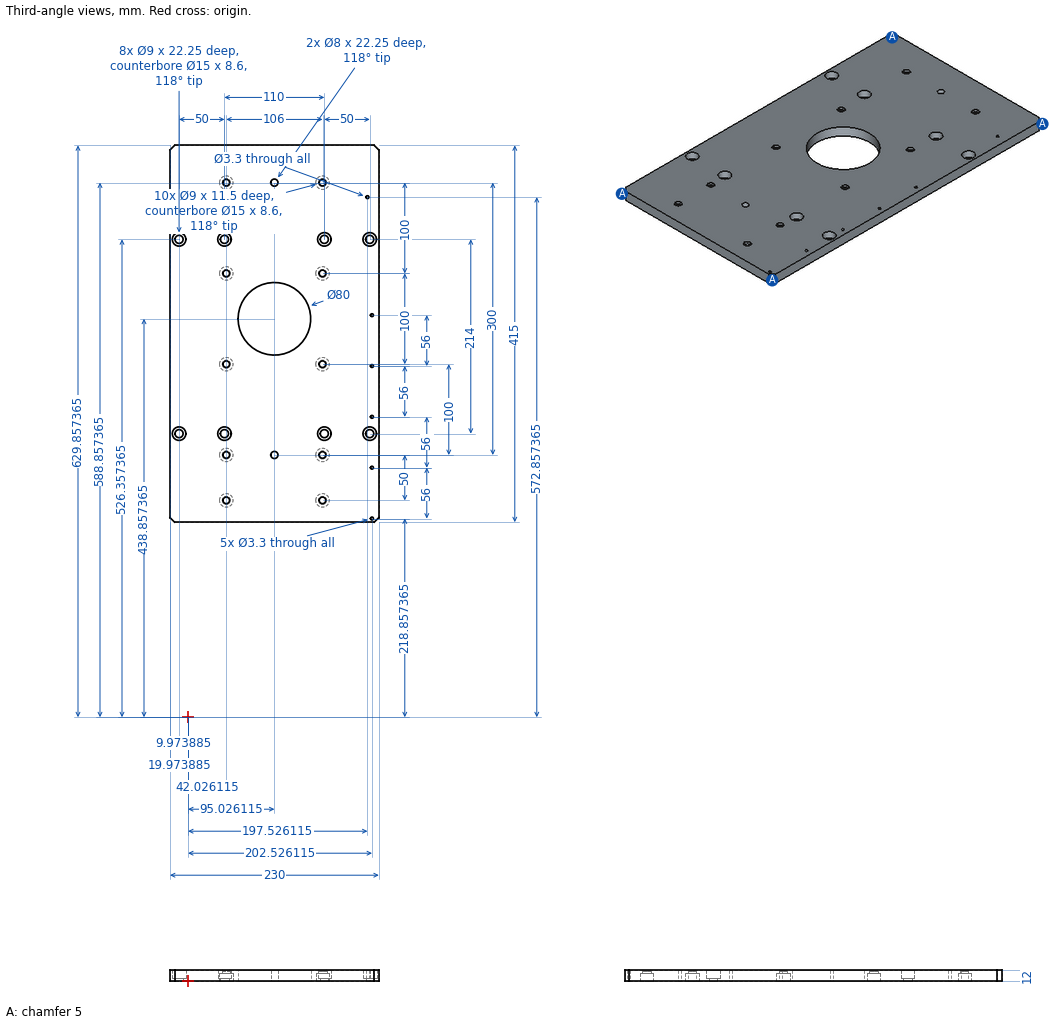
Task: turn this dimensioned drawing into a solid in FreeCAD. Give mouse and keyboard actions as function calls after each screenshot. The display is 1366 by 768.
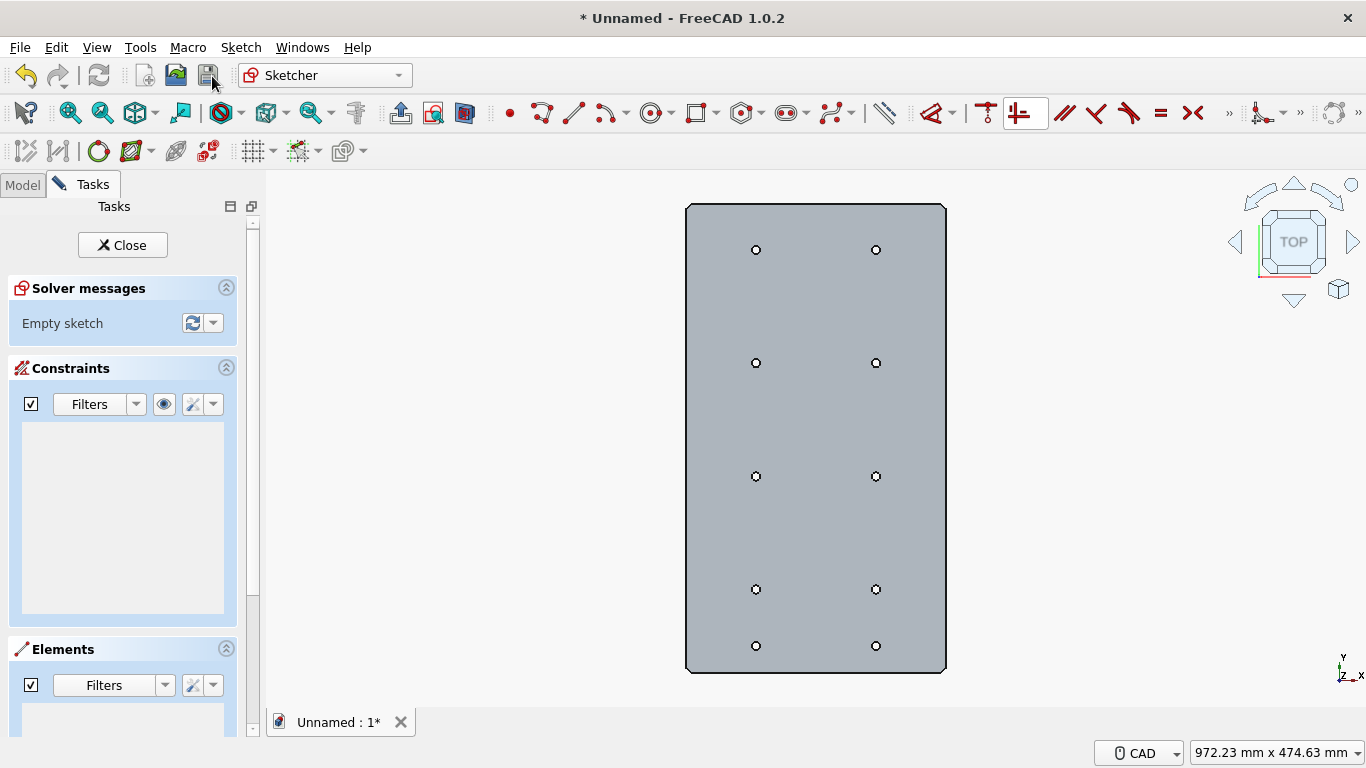
scroll(664, 223, down, 3)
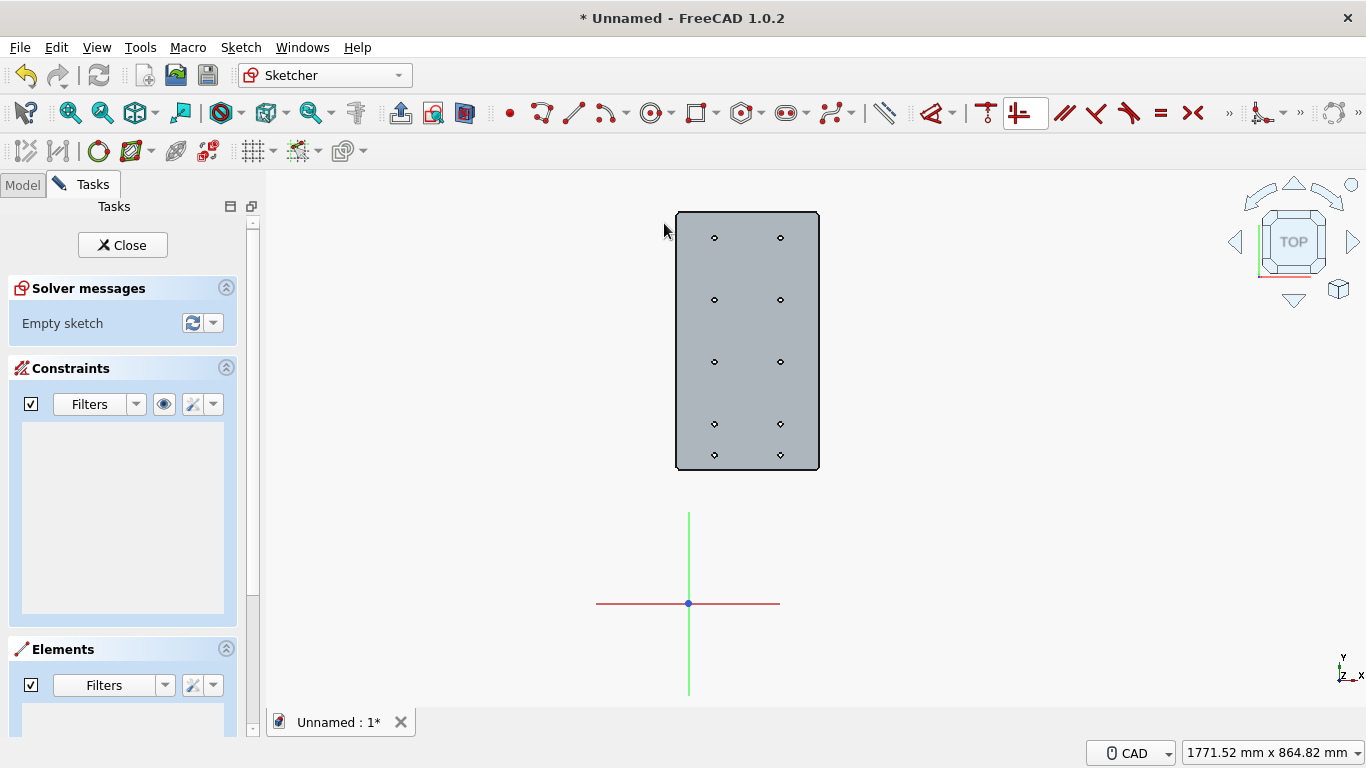
click(652, 114)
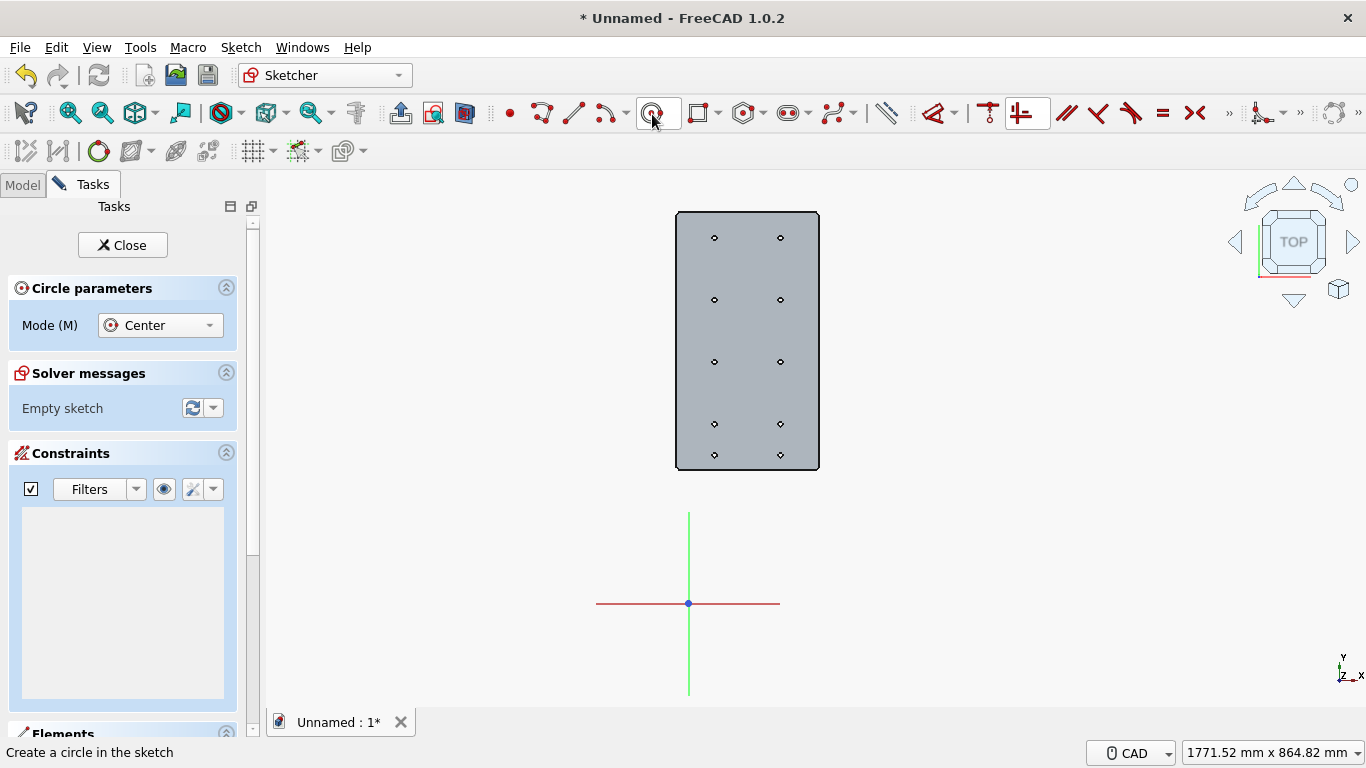
scroll(682, 277, up, 11)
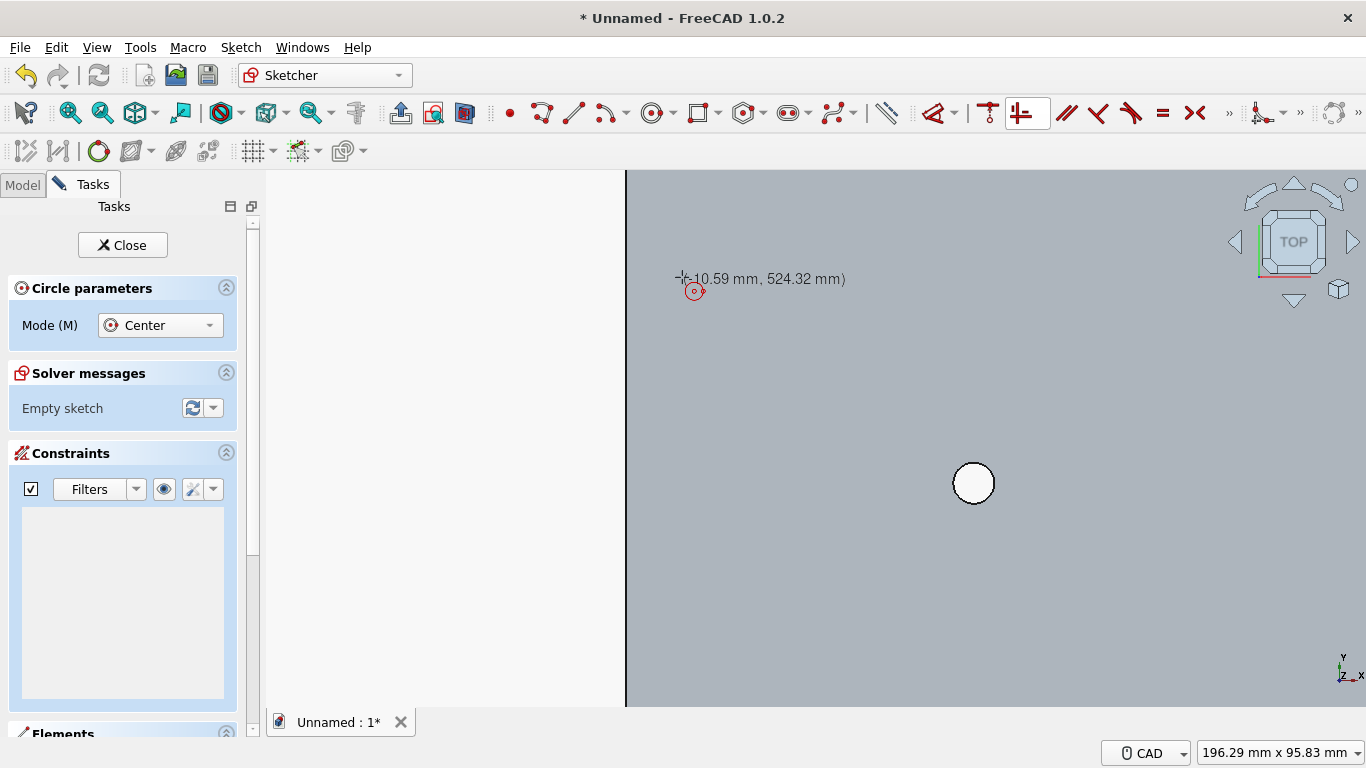
scroll(682, 277, down, 11)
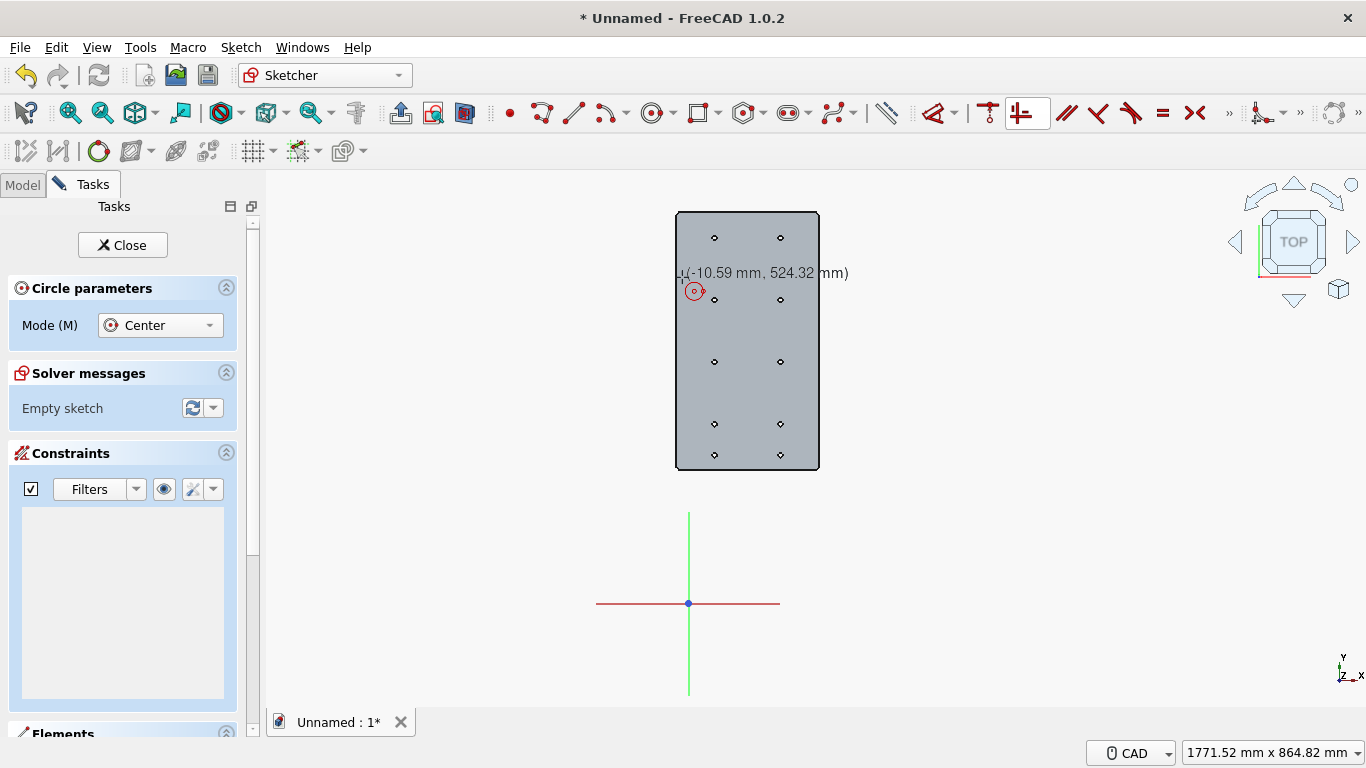
scroll(682, 277, up, 5)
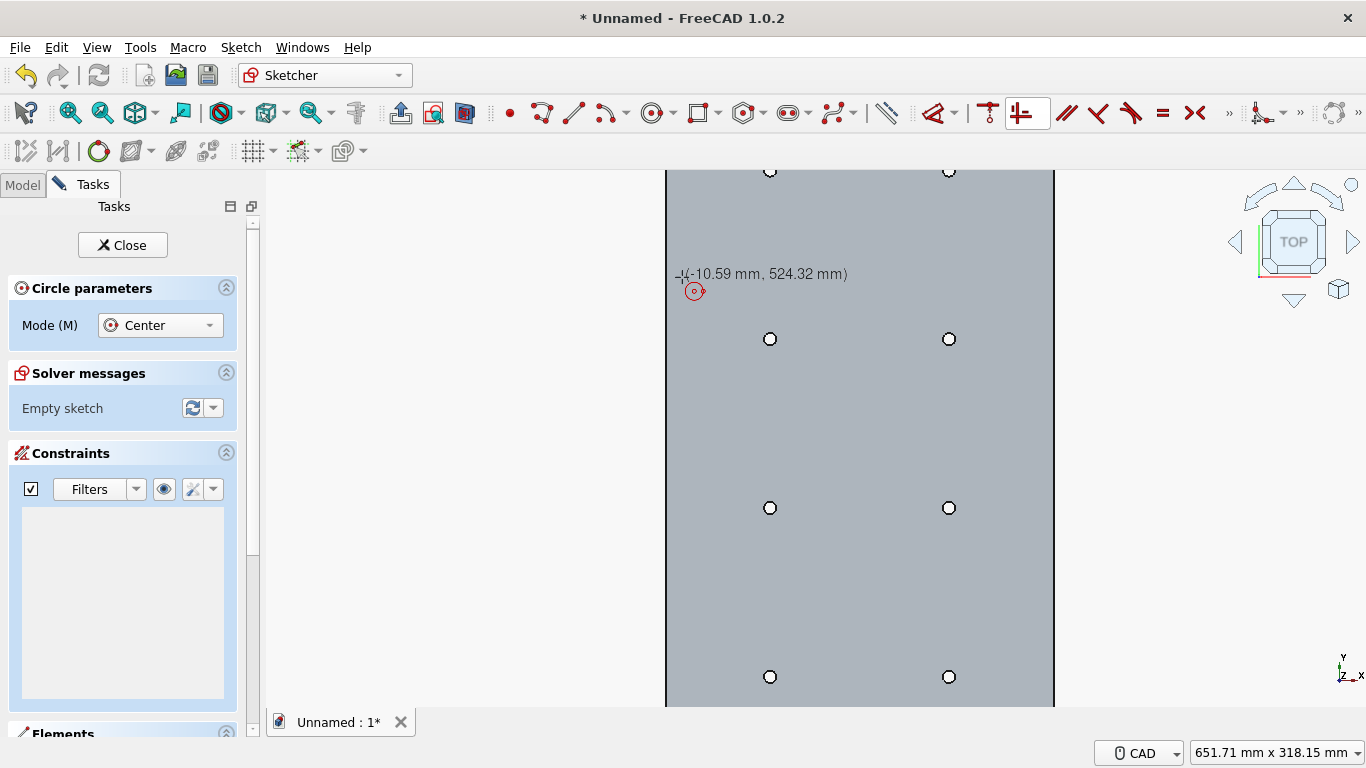
click(682, 276)
move(677, 271)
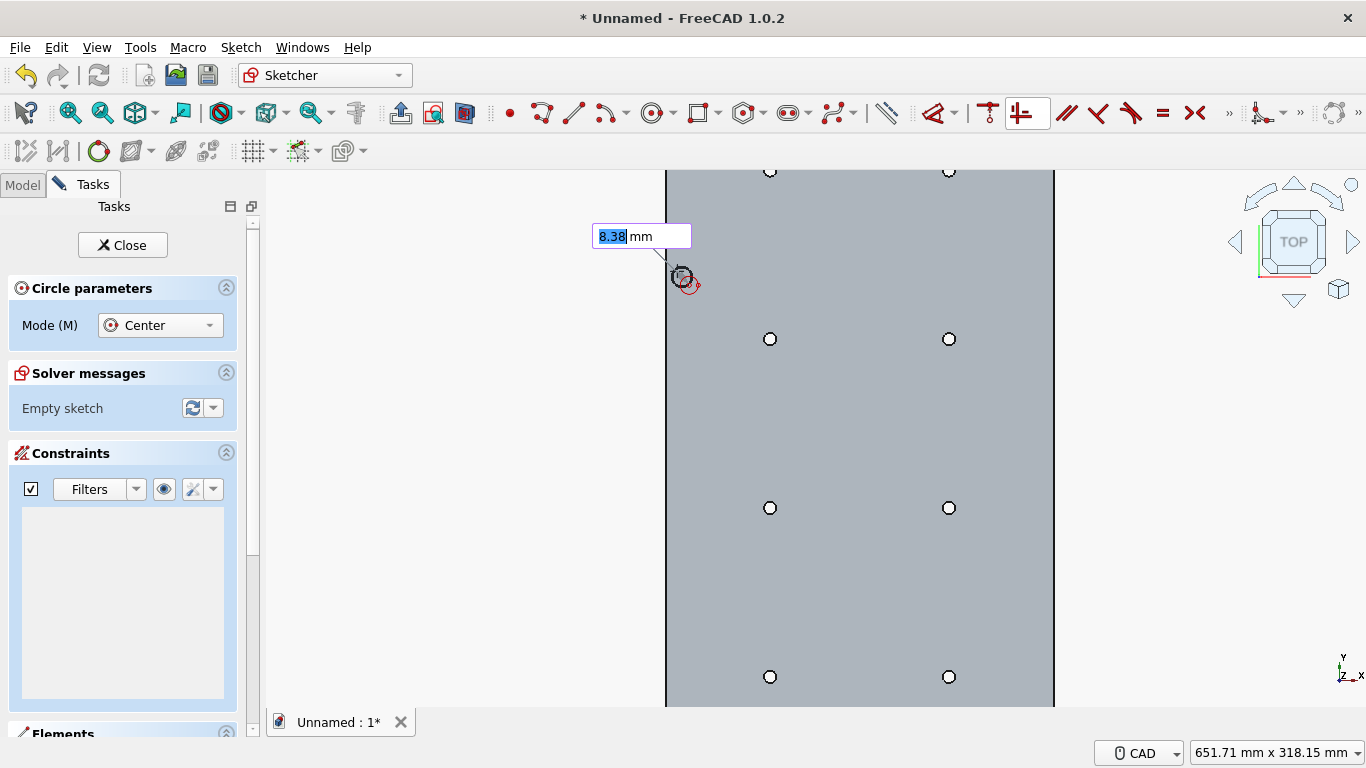
text(9)
key(Return)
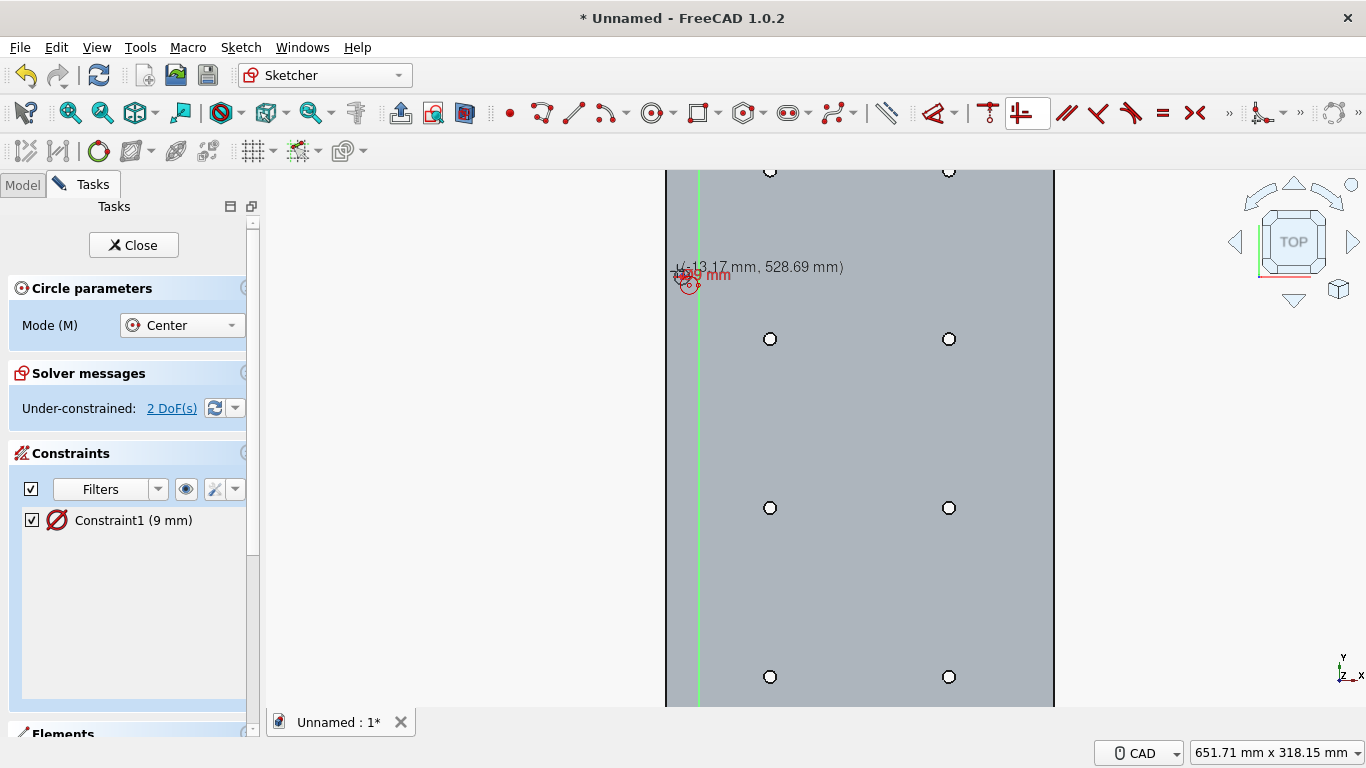
scroll(767, 276, up, 6)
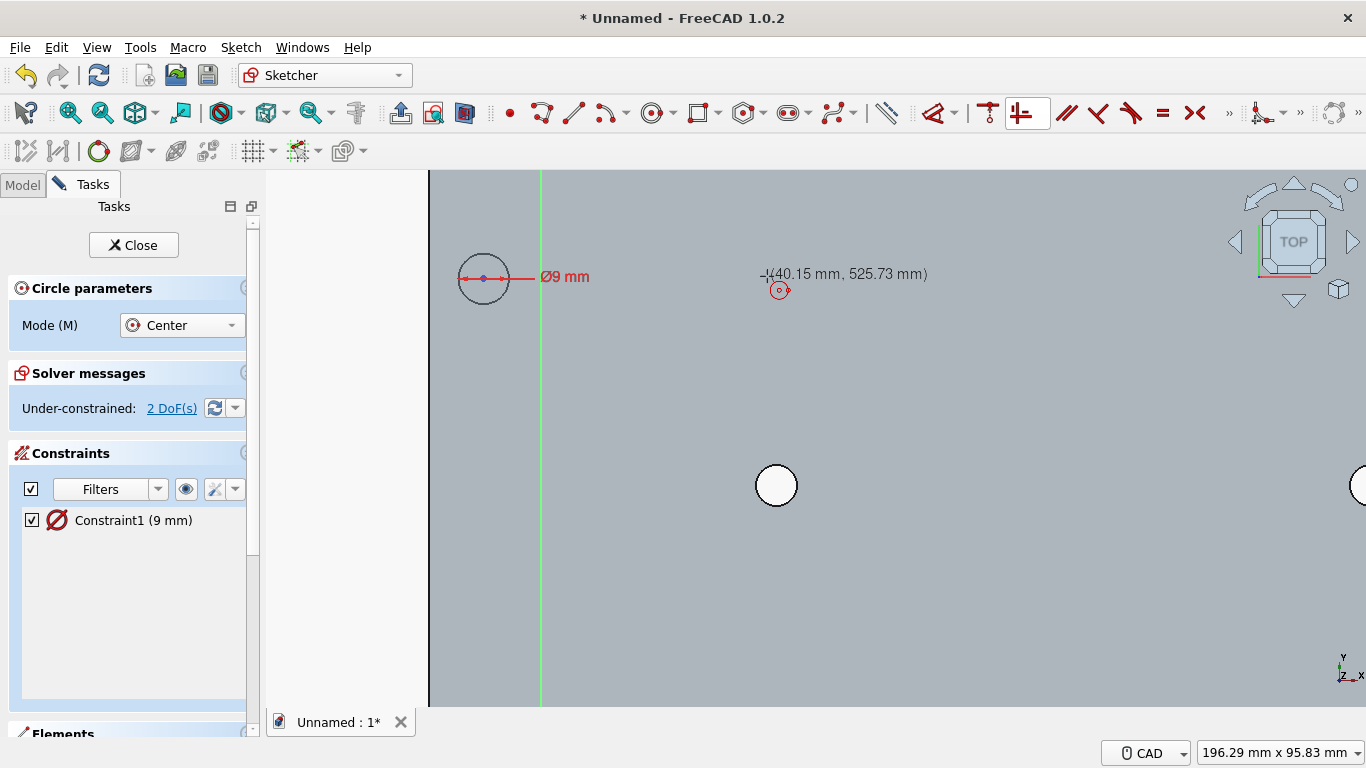
scroll(707, 277, down, 11)